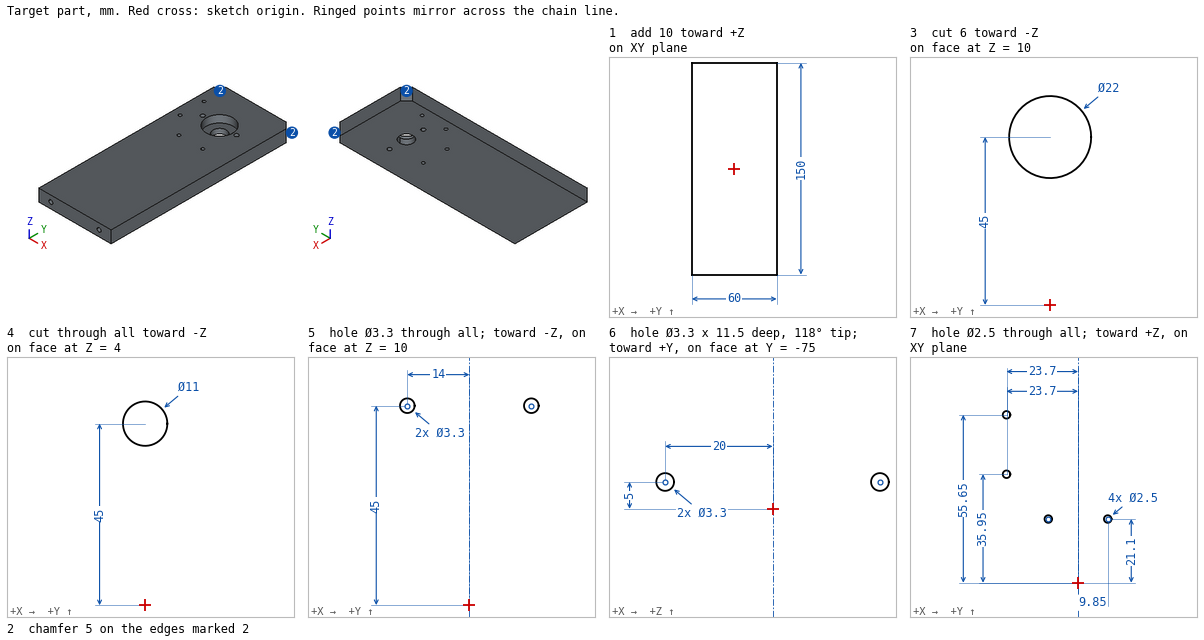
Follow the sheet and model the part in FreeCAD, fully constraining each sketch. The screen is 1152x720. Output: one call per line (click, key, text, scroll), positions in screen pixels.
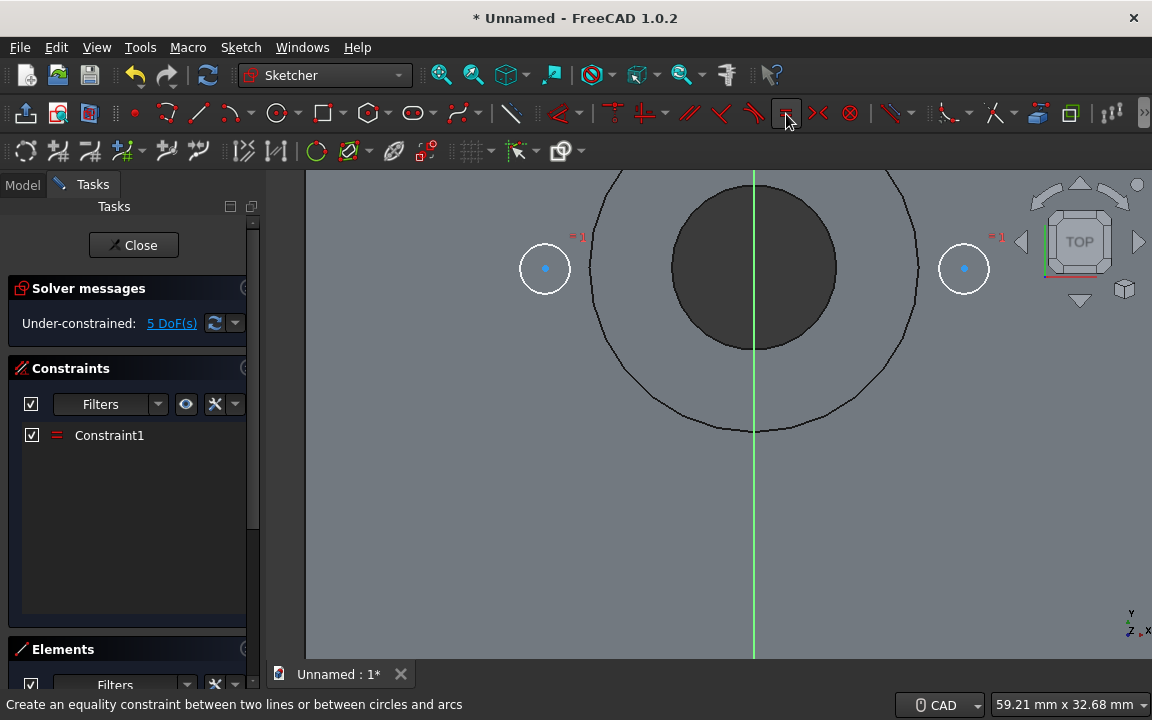
click(545, 269)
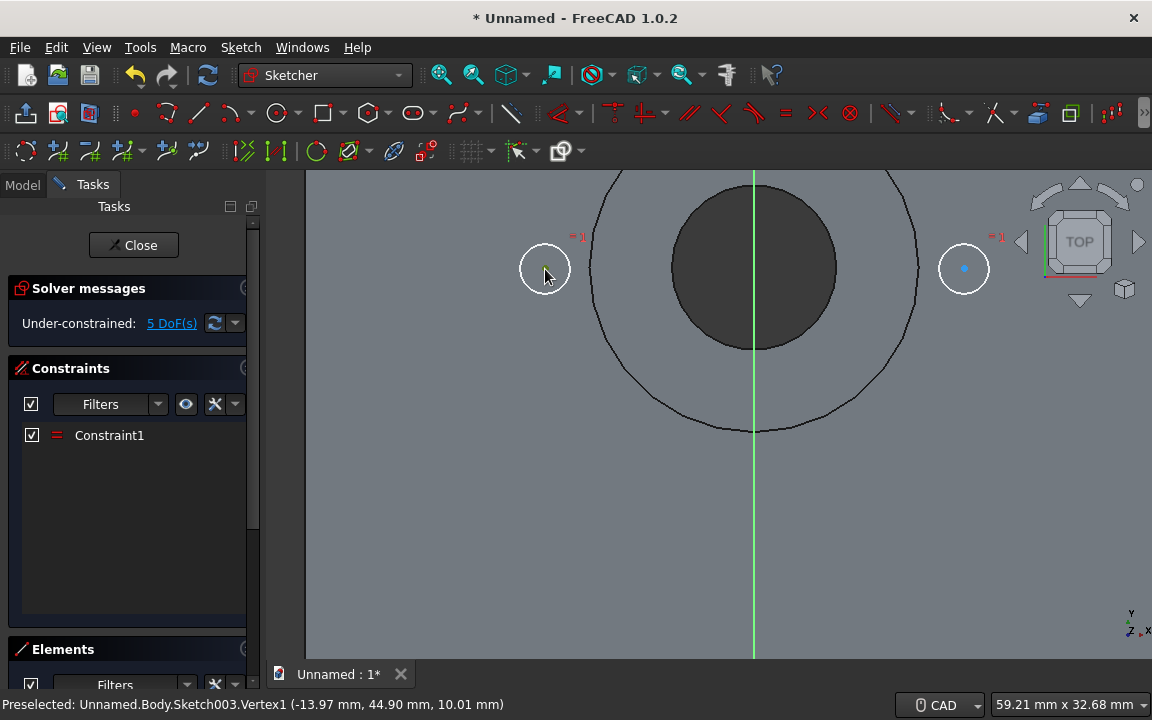
click(964, 269)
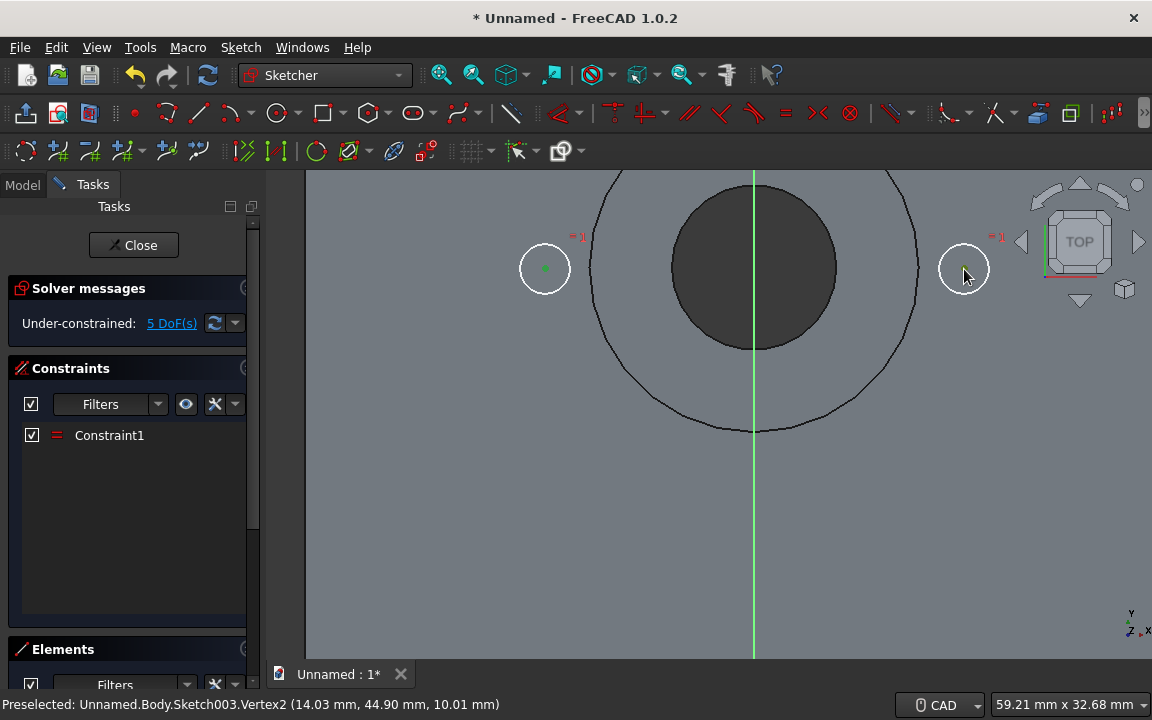
click(754, 600)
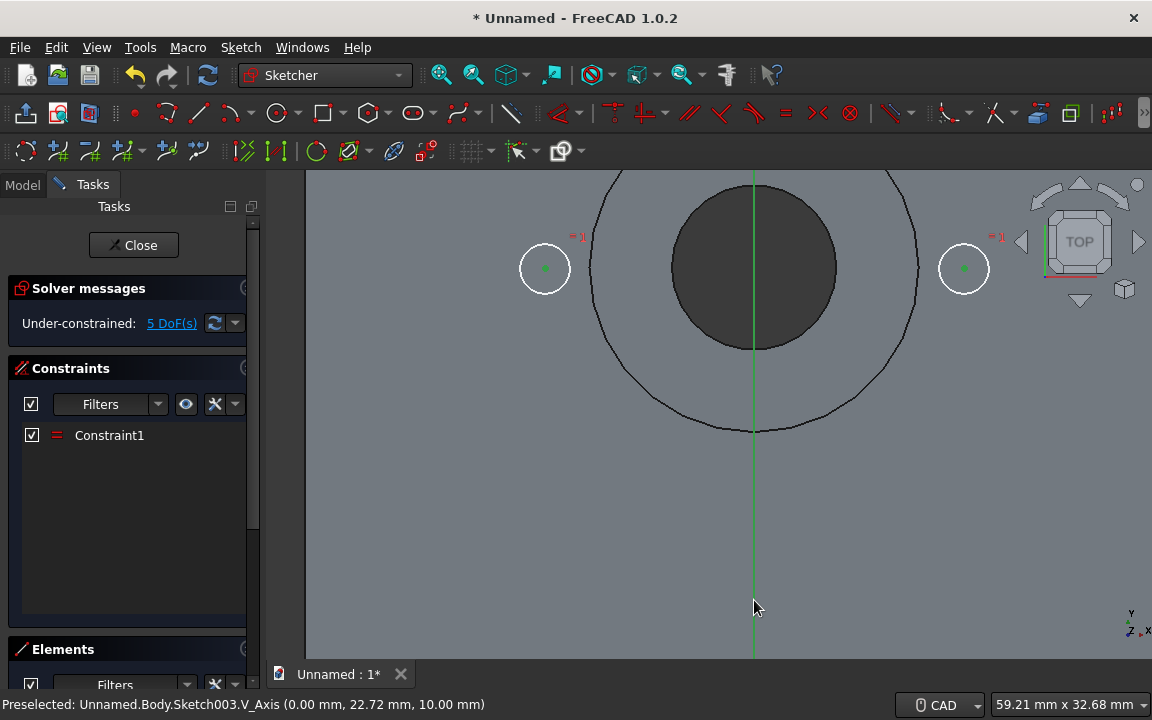
click(818, 114)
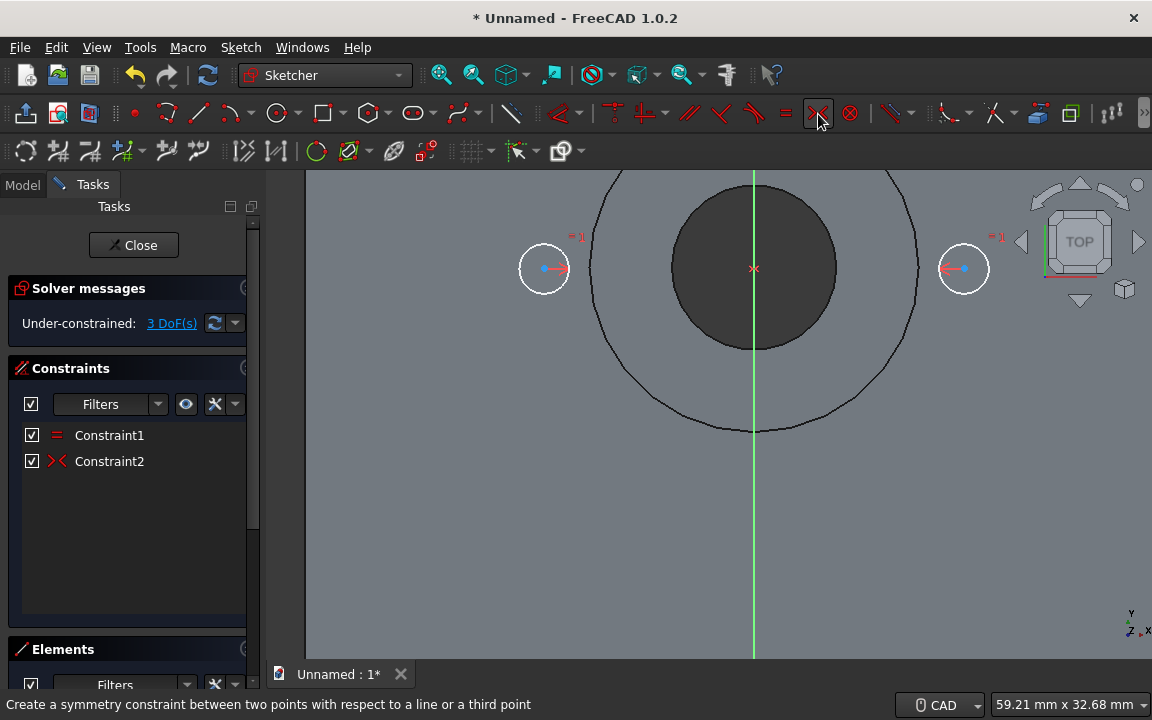
click(558, 114)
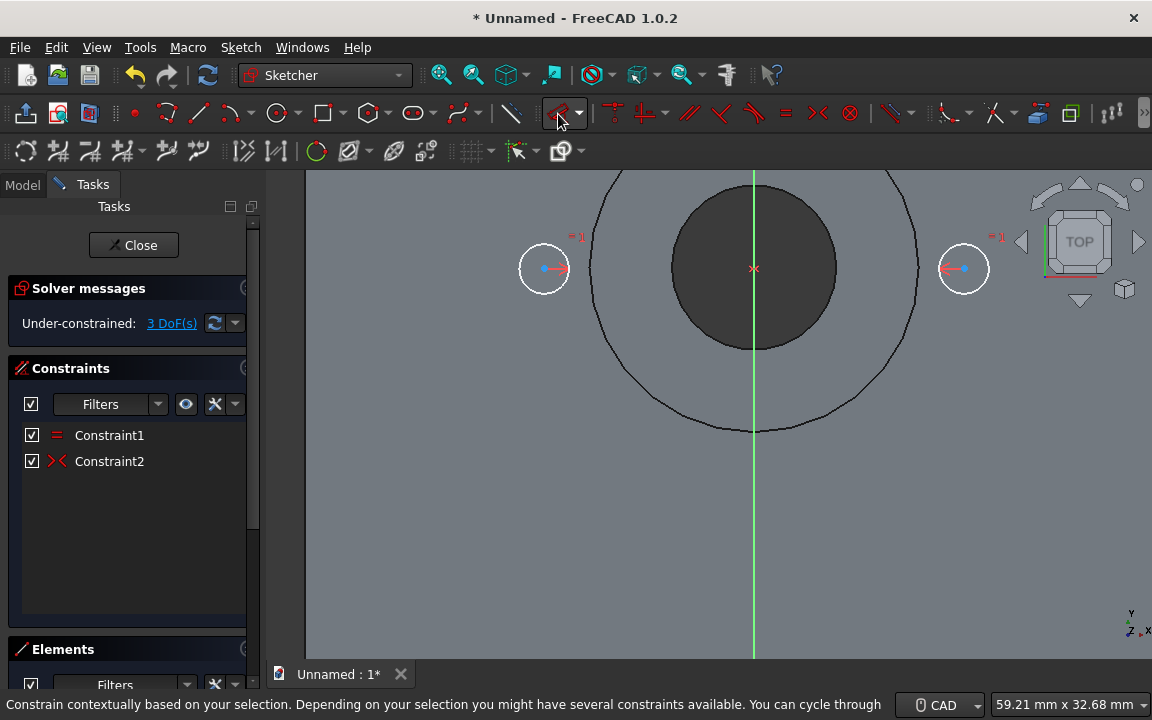
click(562, 251)
click(585, 228)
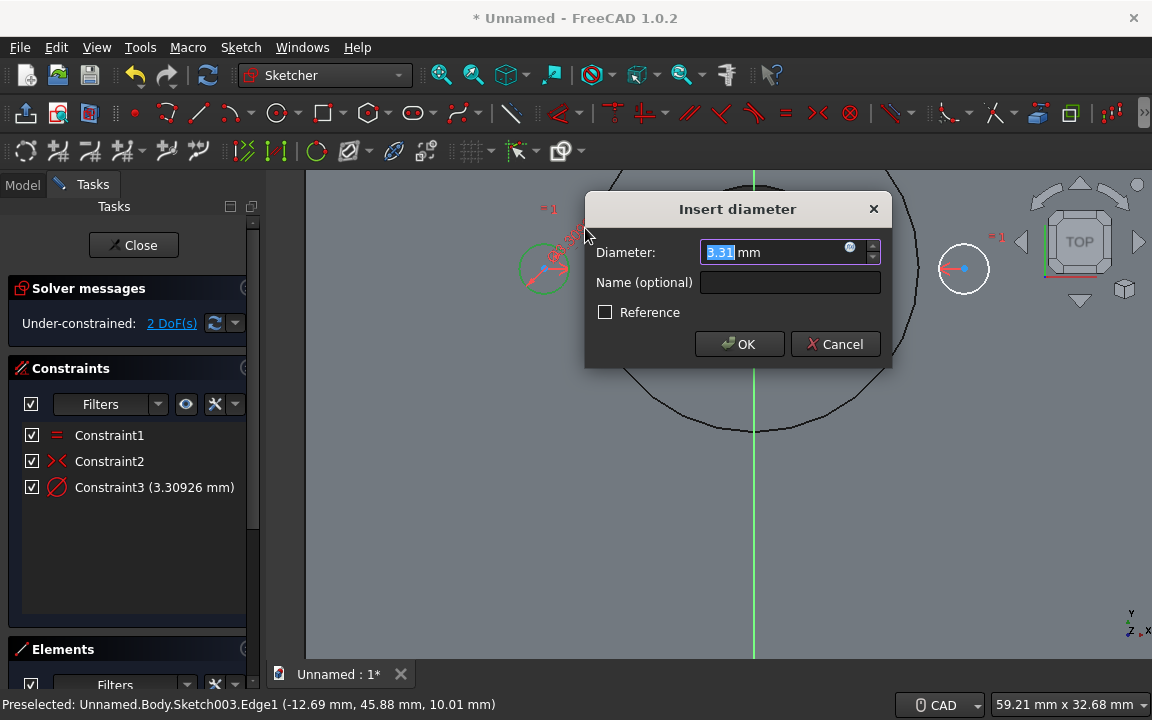
text(3.3)
key(Return)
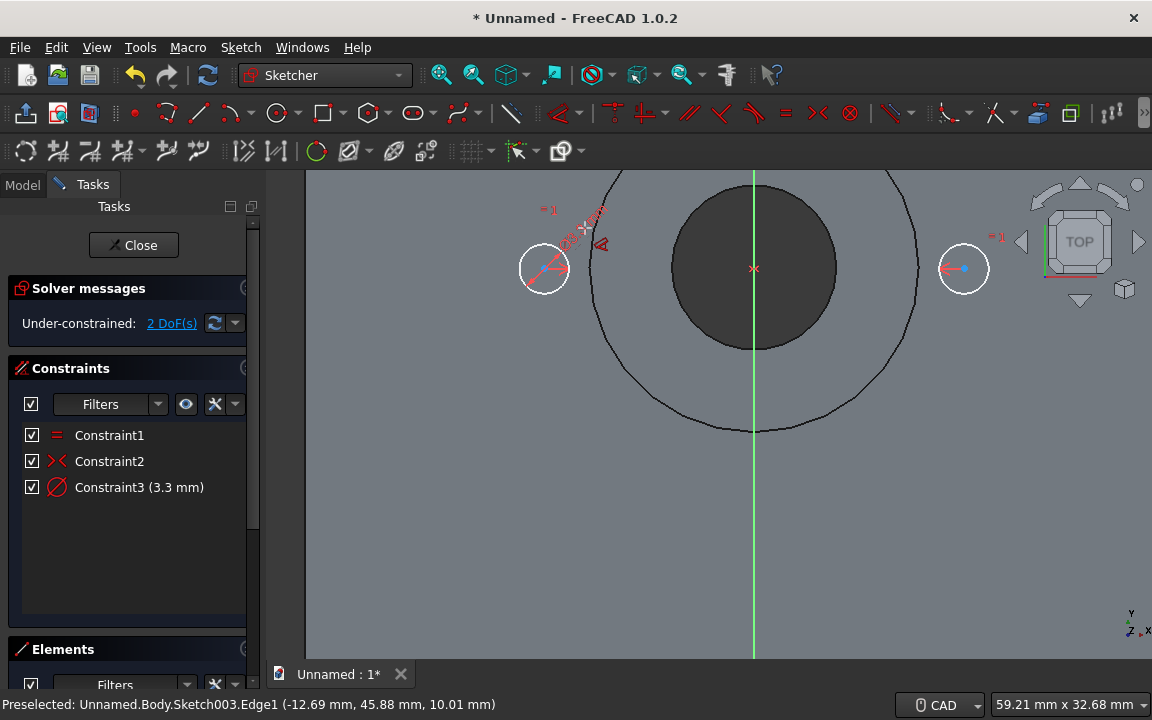
click(544, 269)
click(697, 235)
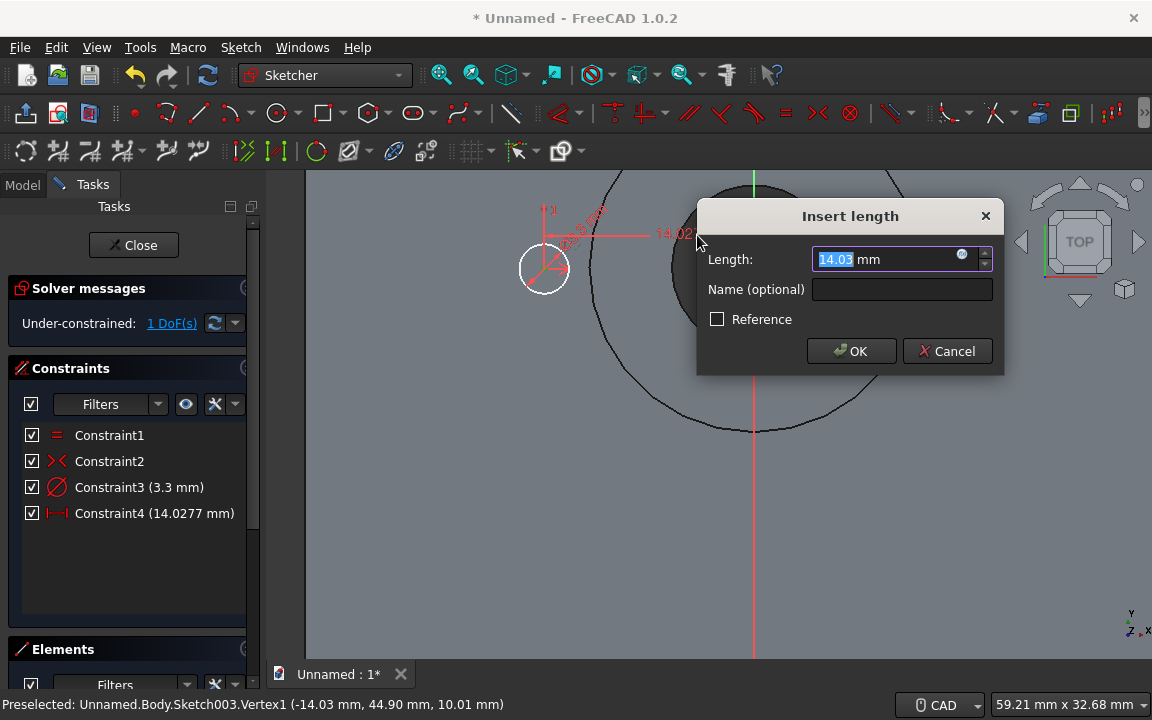
text(14)
key(Return)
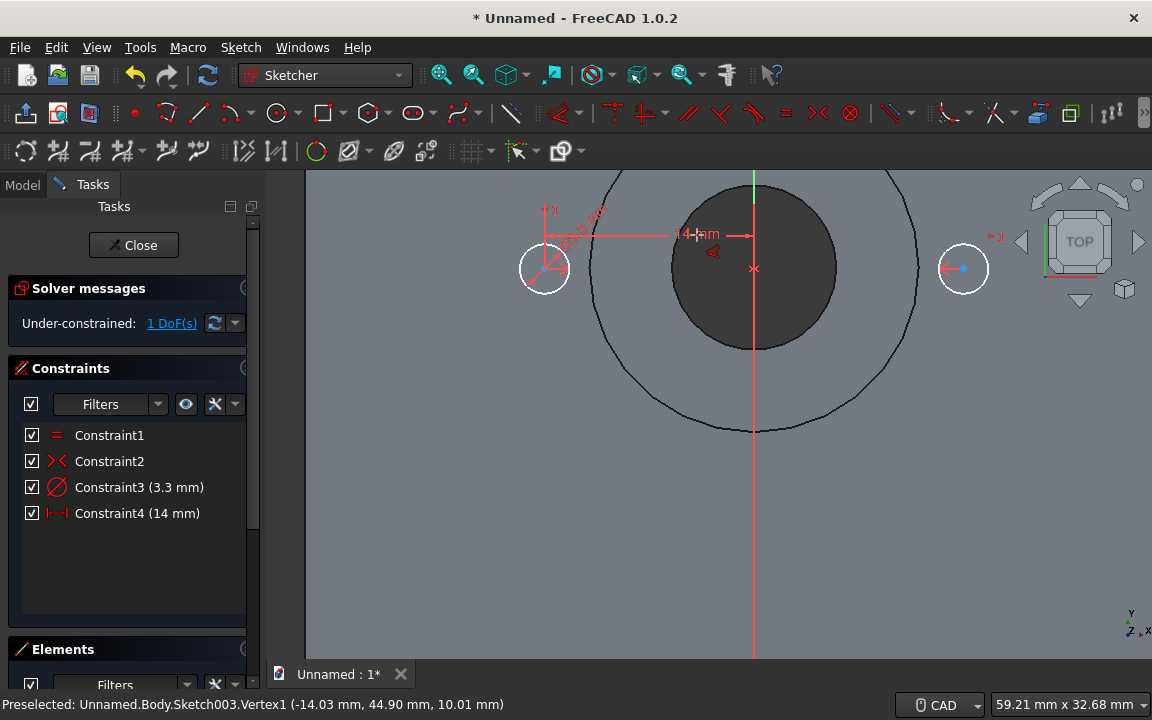
click(545, 269)
click(511, 450)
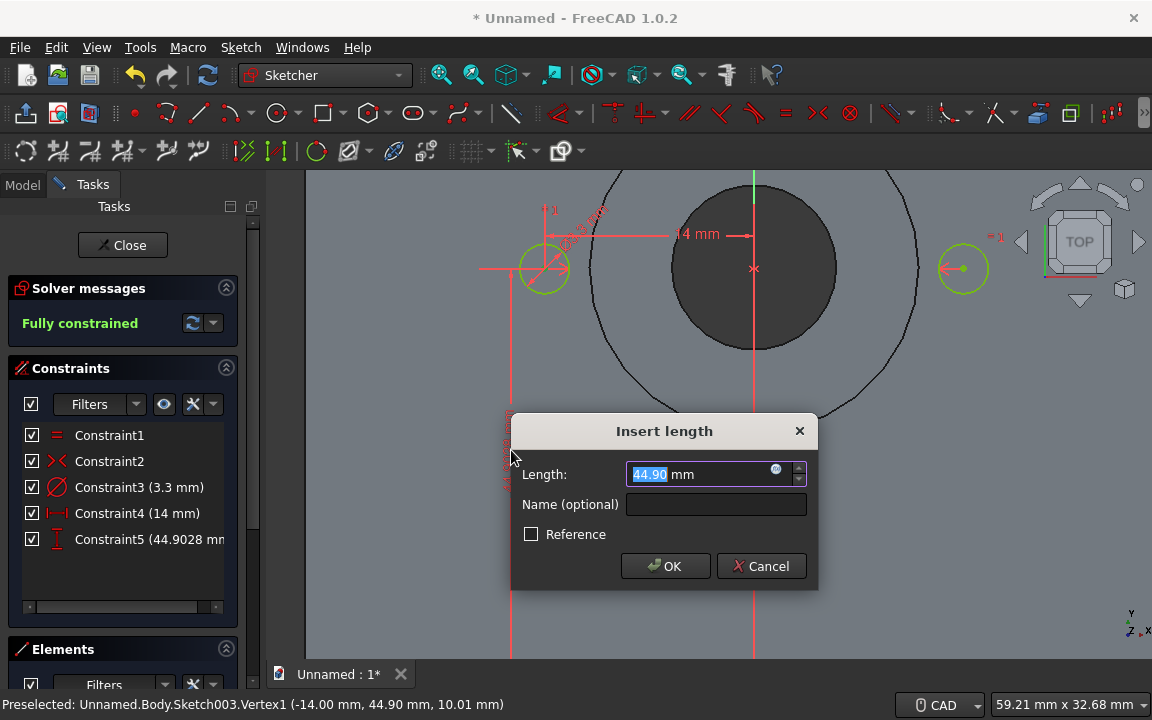
text(45)
key(Return)
key(Escape)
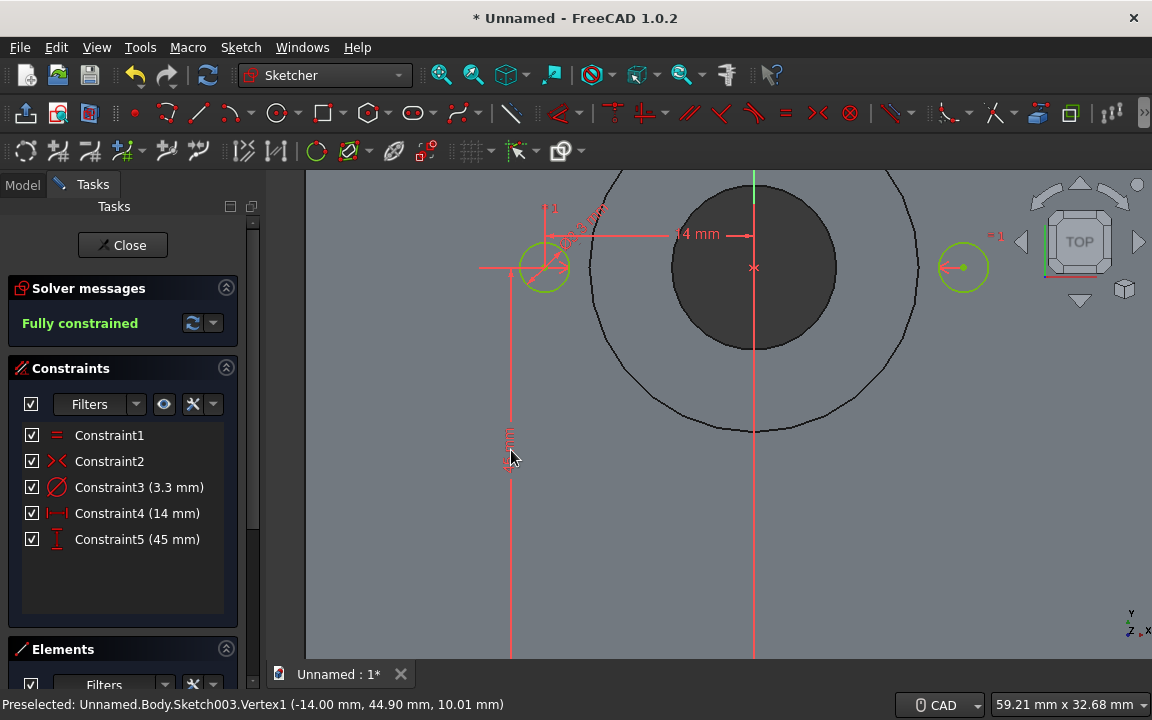
click(123, 245)